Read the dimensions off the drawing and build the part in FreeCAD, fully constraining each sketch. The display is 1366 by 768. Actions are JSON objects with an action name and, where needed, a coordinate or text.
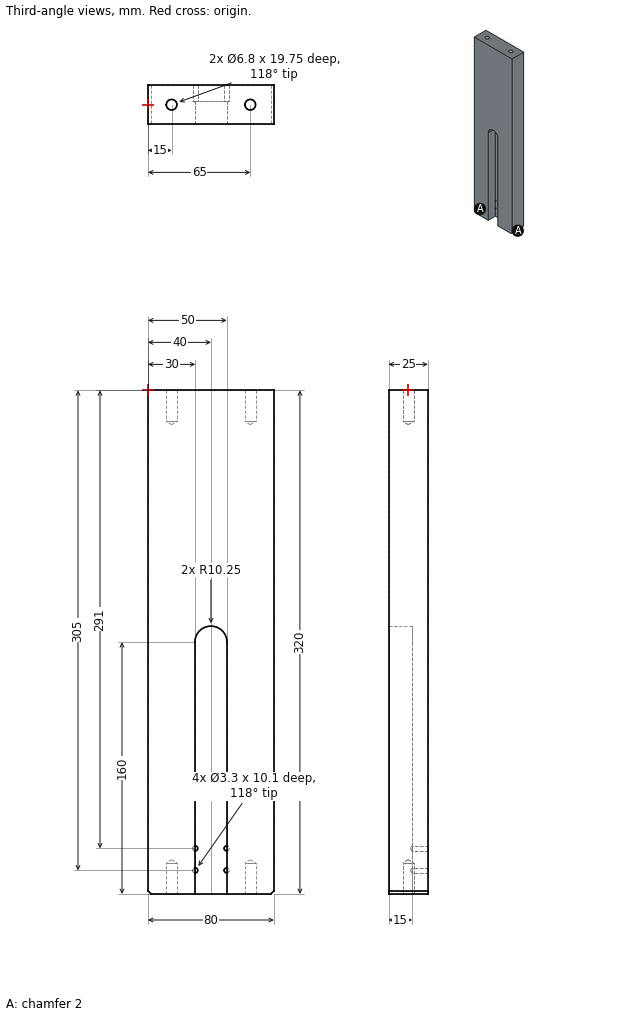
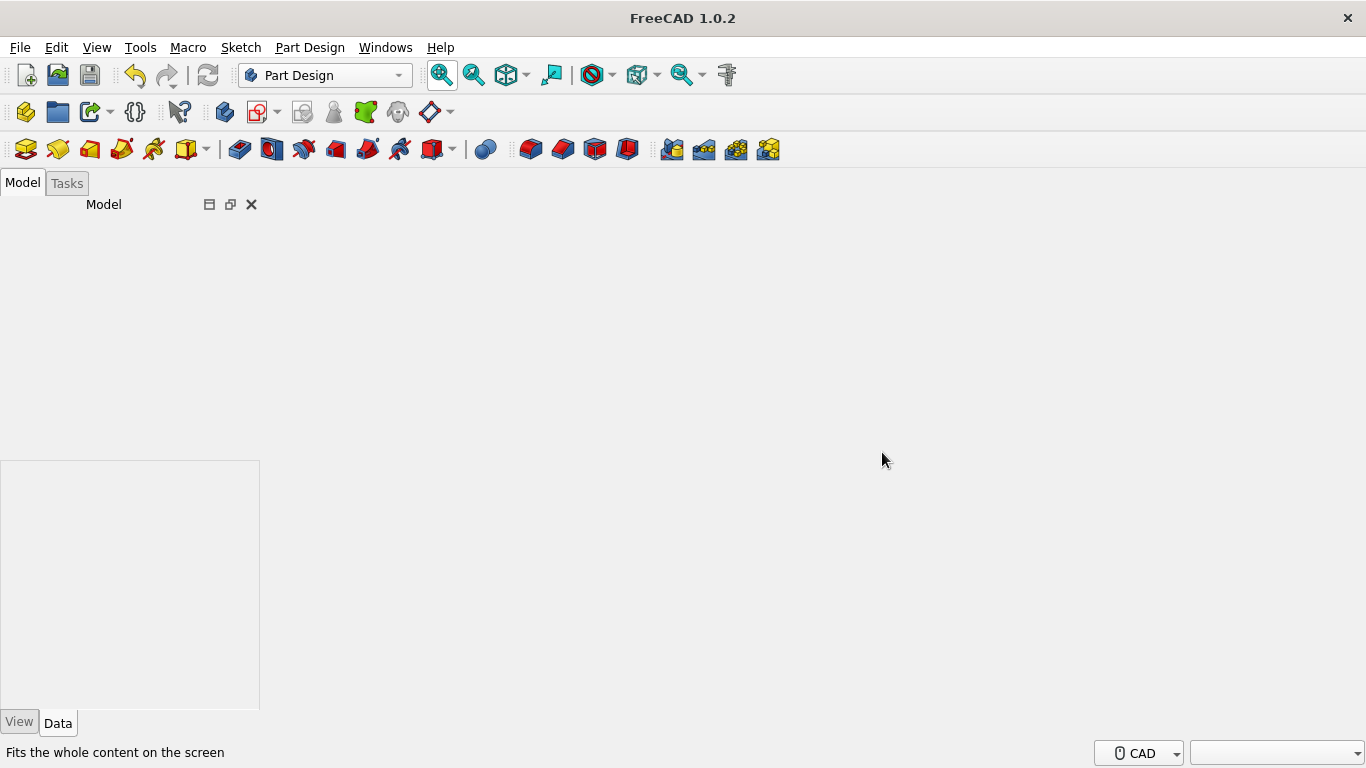
{"action": "key", "text": "ctrl+n"}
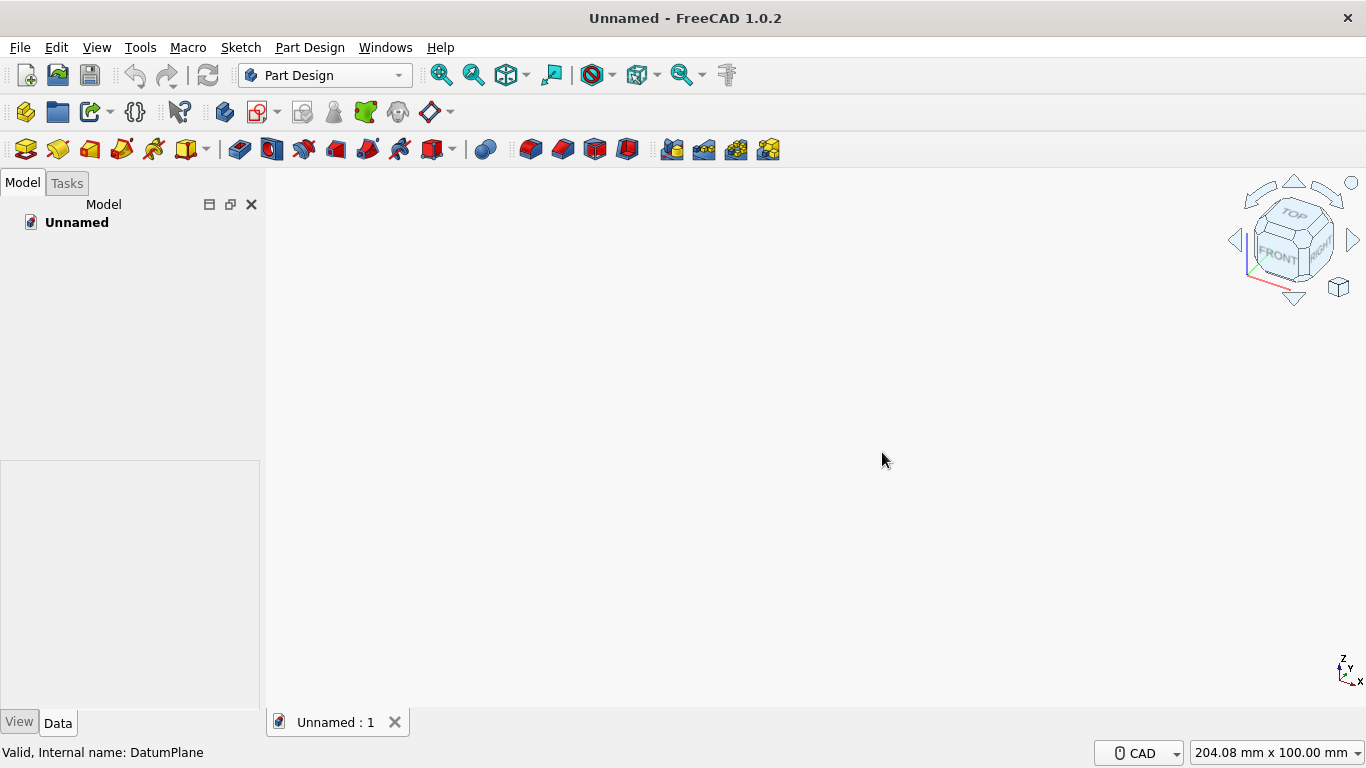
{"action": "left_click", "coordinate": [258, 112]}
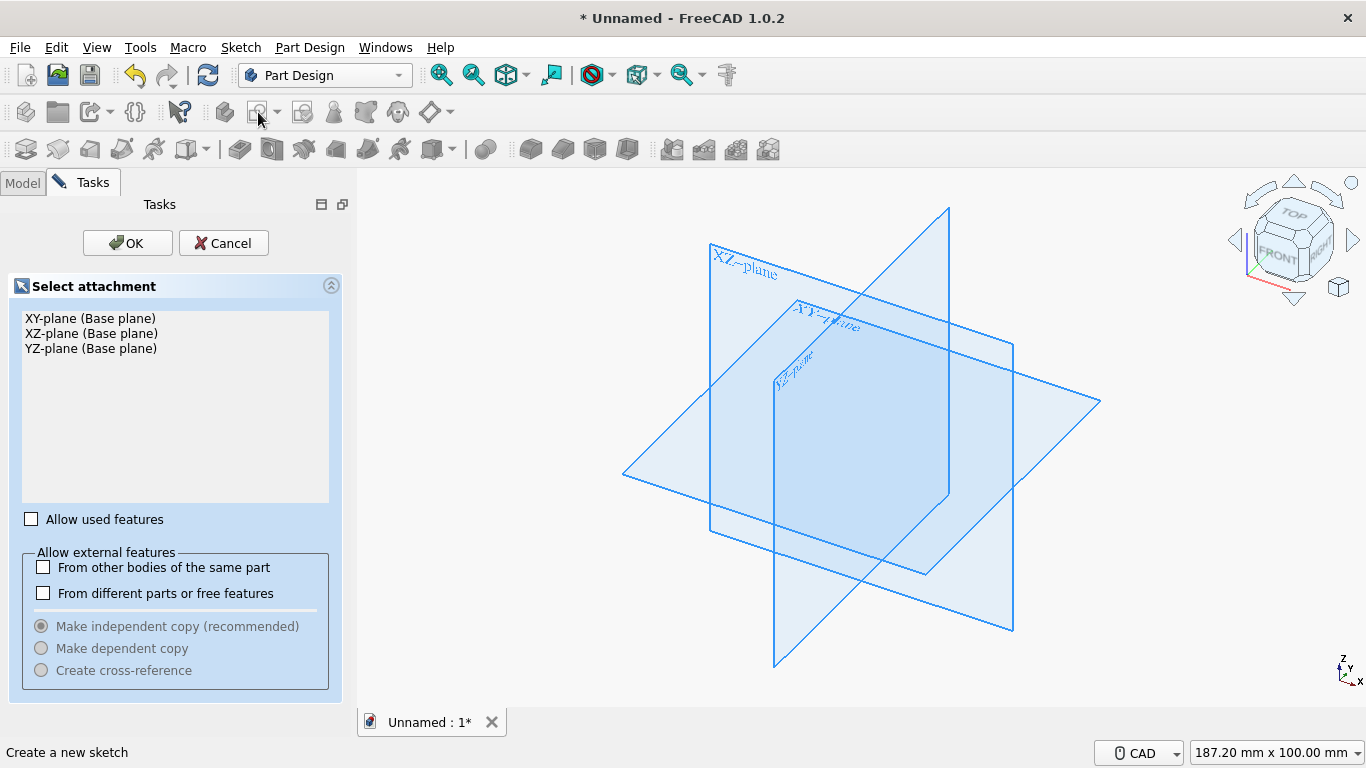
{"action": "left_click", "coordinate": [82, 334]}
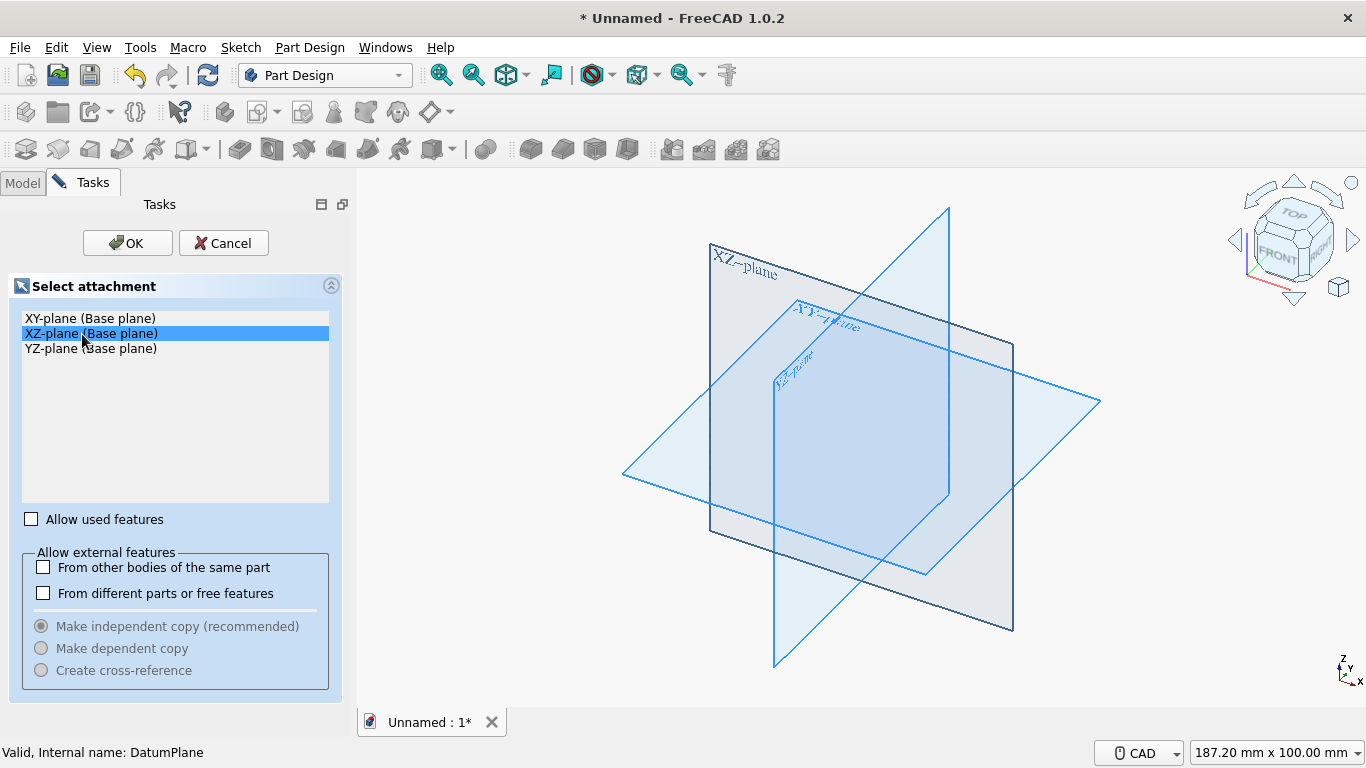
{"action": "left_click", "coordinate": [128, 243]}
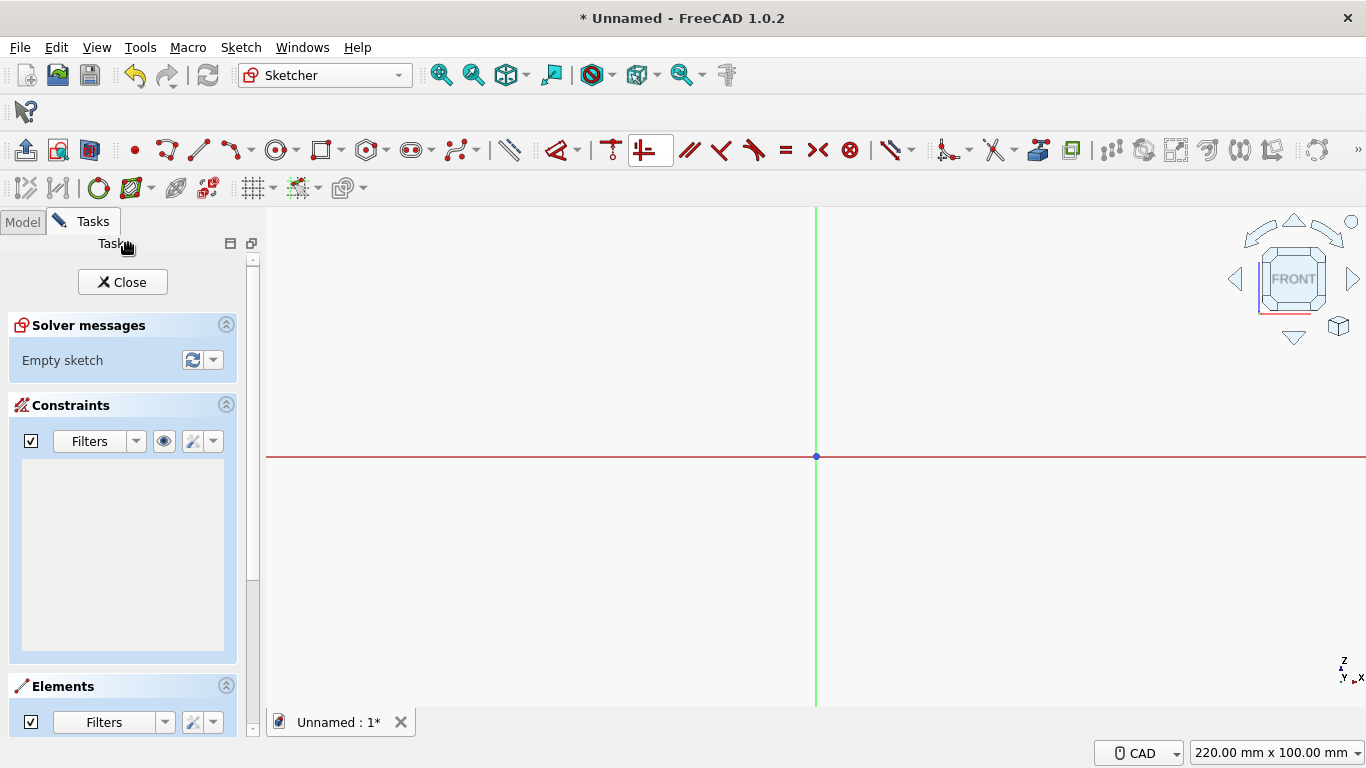
{"action": "scroll", "coordinate": [680, 255], "scroll_direction": "down", "scroll_amount": 8}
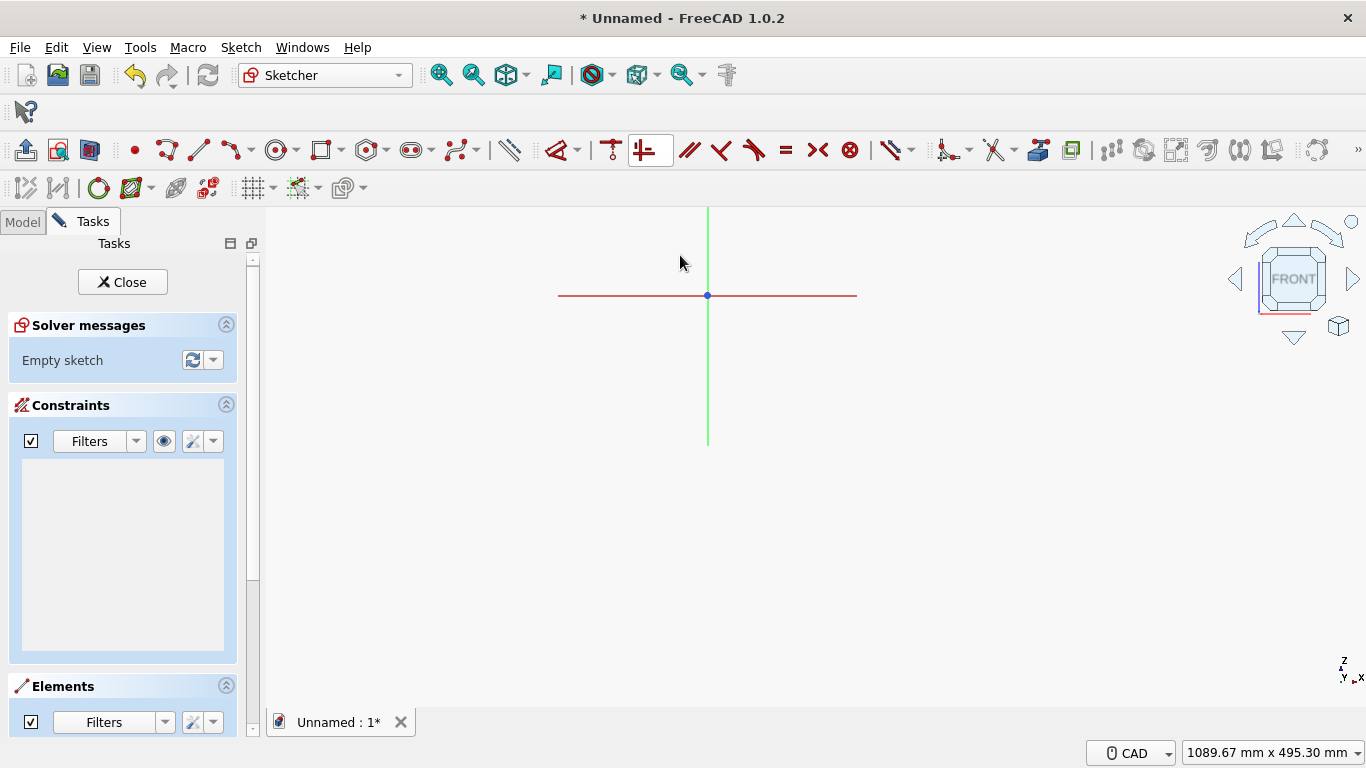
{"action": "left_click", "coordinate": [322, 150]}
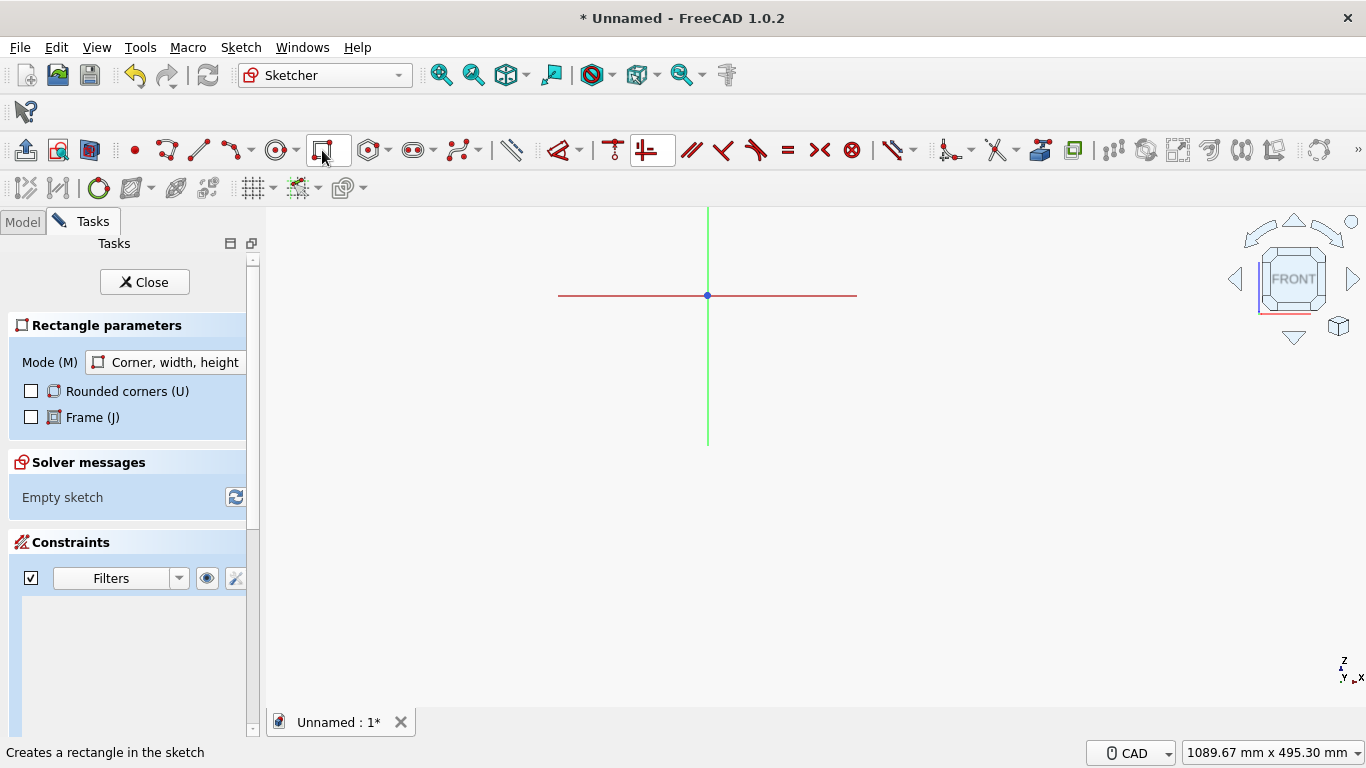
{"action": "left_click", "coordinate": [708, 296]}
{"action": "mouse_move", "coordinate": [789, 619]}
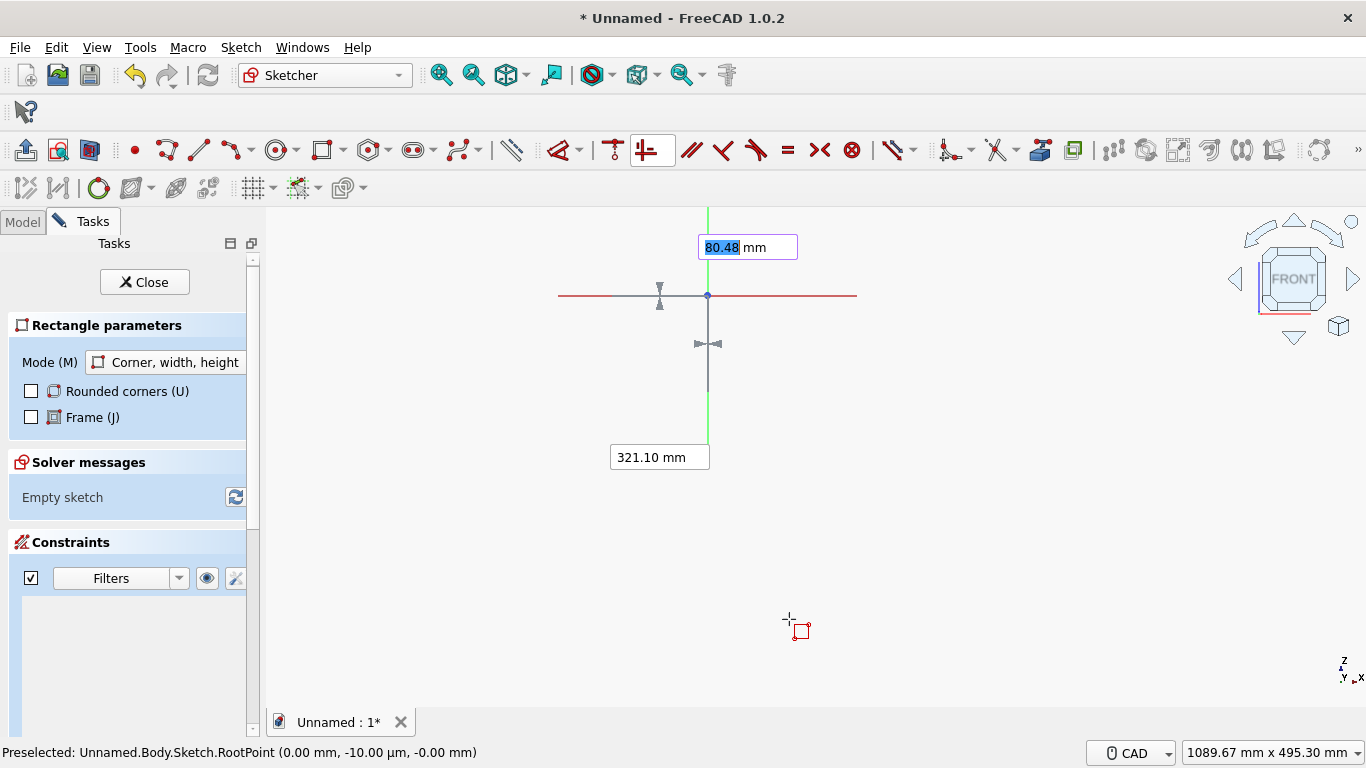
{"action": "type", "text": "80"}
{"action": "key", "text": "Tab"}
{"action": "type", "text": "320"}
{"action": "key", "text": "Return"}
{"action": "key", "text": "Escape"}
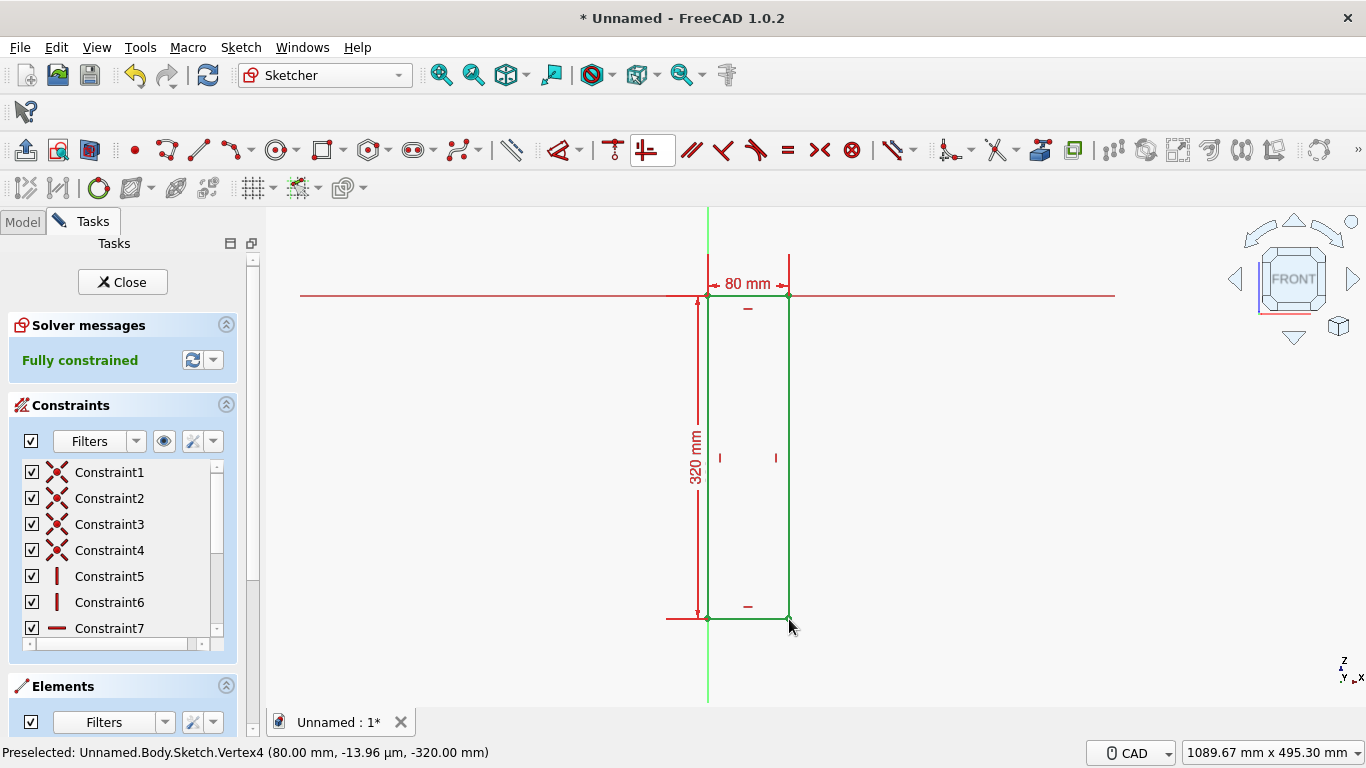
{"action": "left_click", "coordinate": [123, 282]}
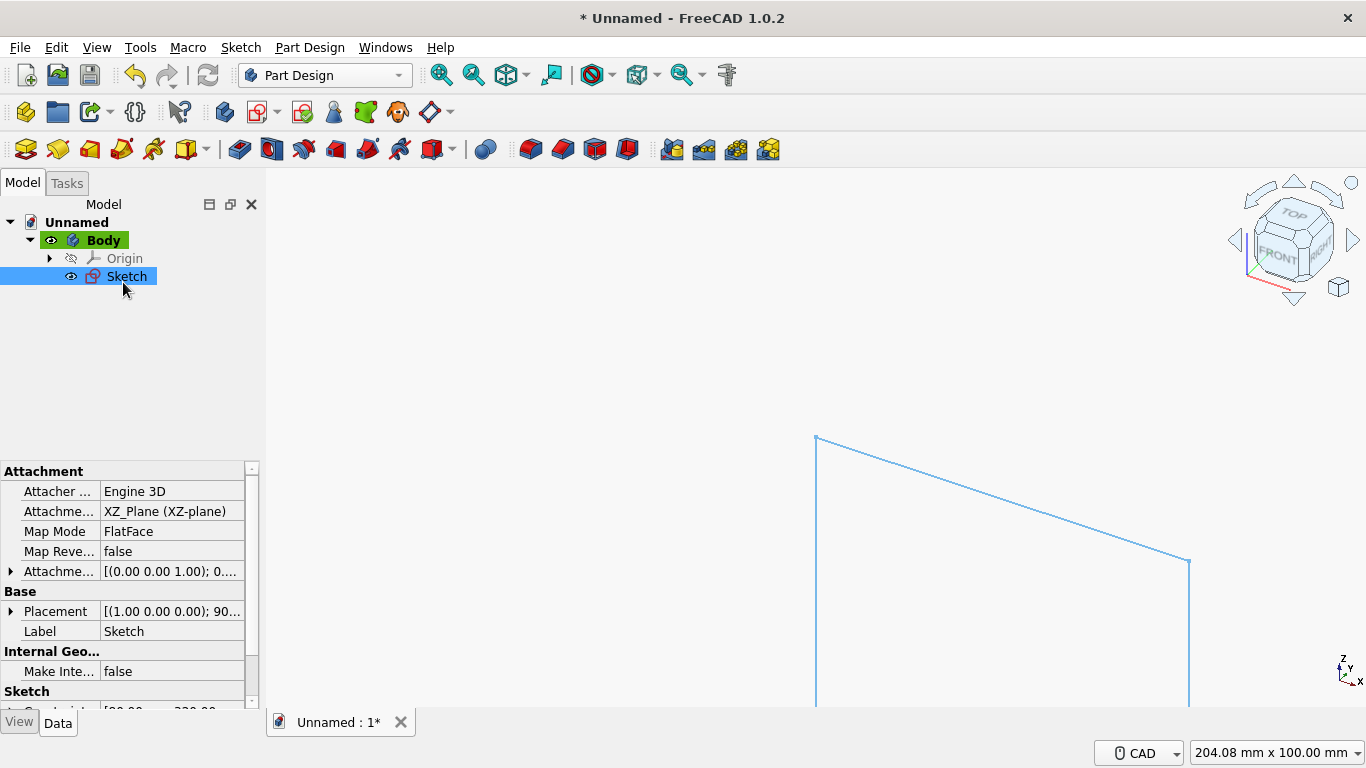
{"action": "left_click", "coordinate": [26, 150]}